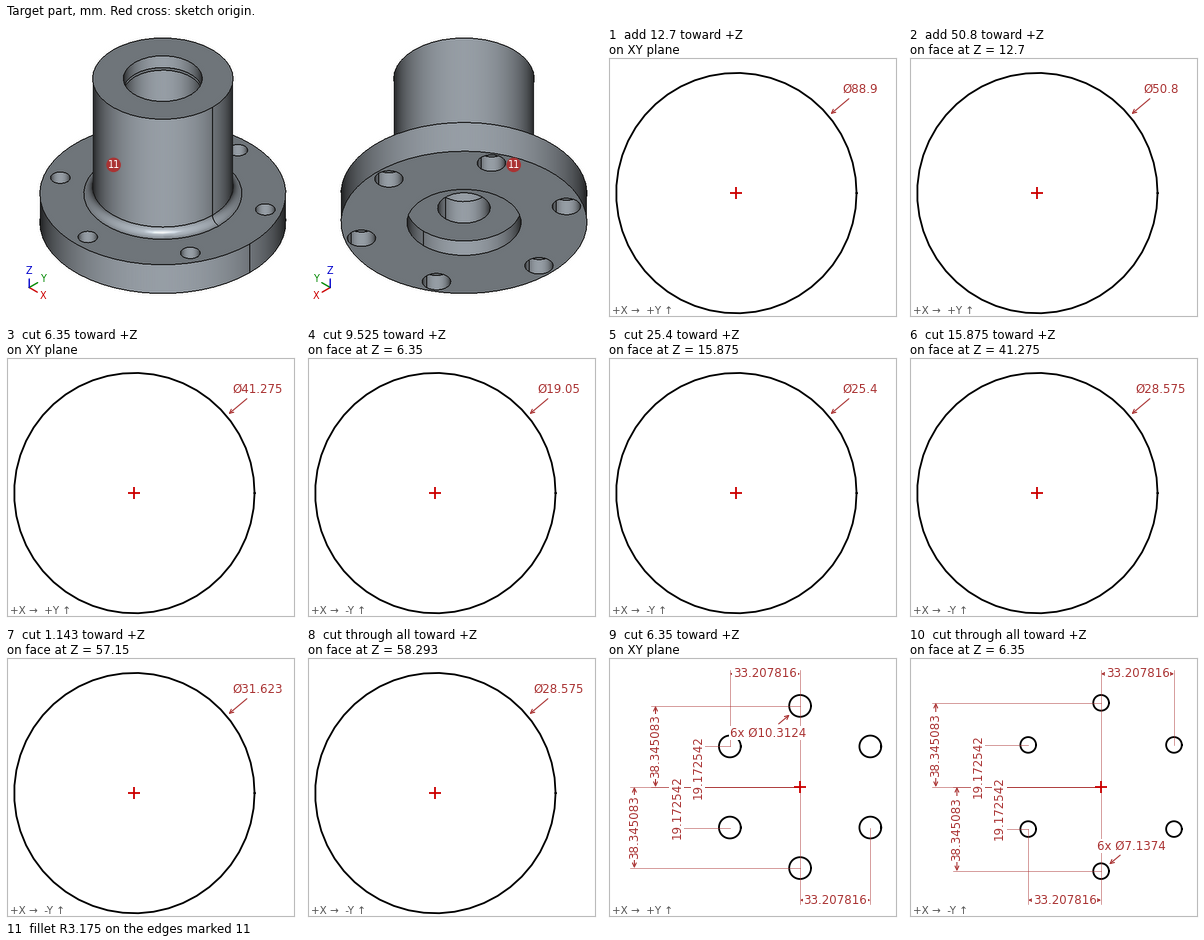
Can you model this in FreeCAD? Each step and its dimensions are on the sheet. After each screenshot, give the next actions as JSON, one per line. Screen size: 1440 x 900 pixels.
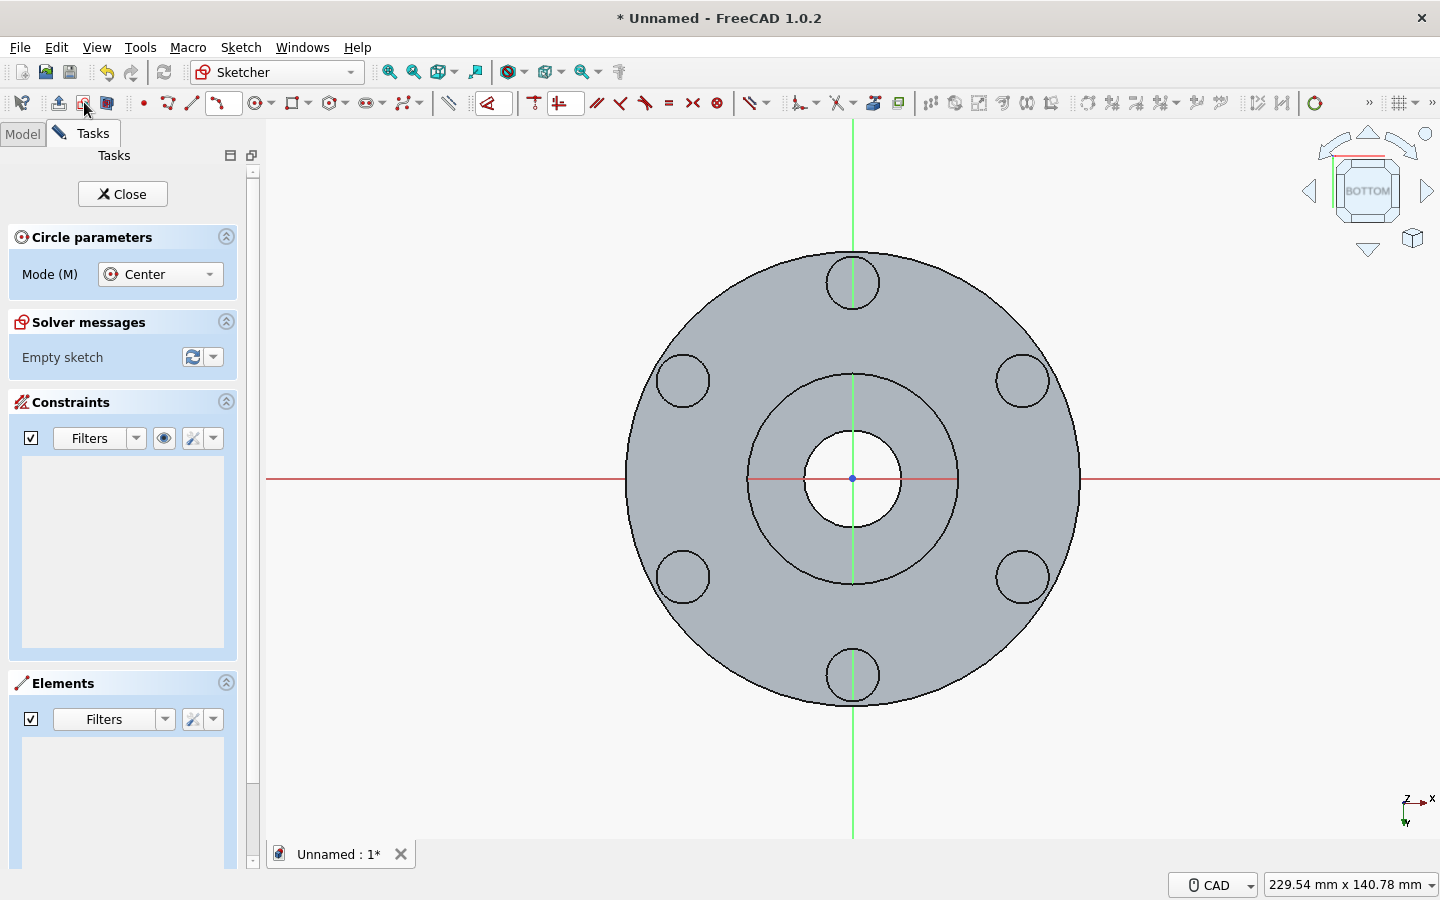
{"action": "scroll", "coordinate": [853, 675], "scroll_direction": "up", "scroll_amount": 2}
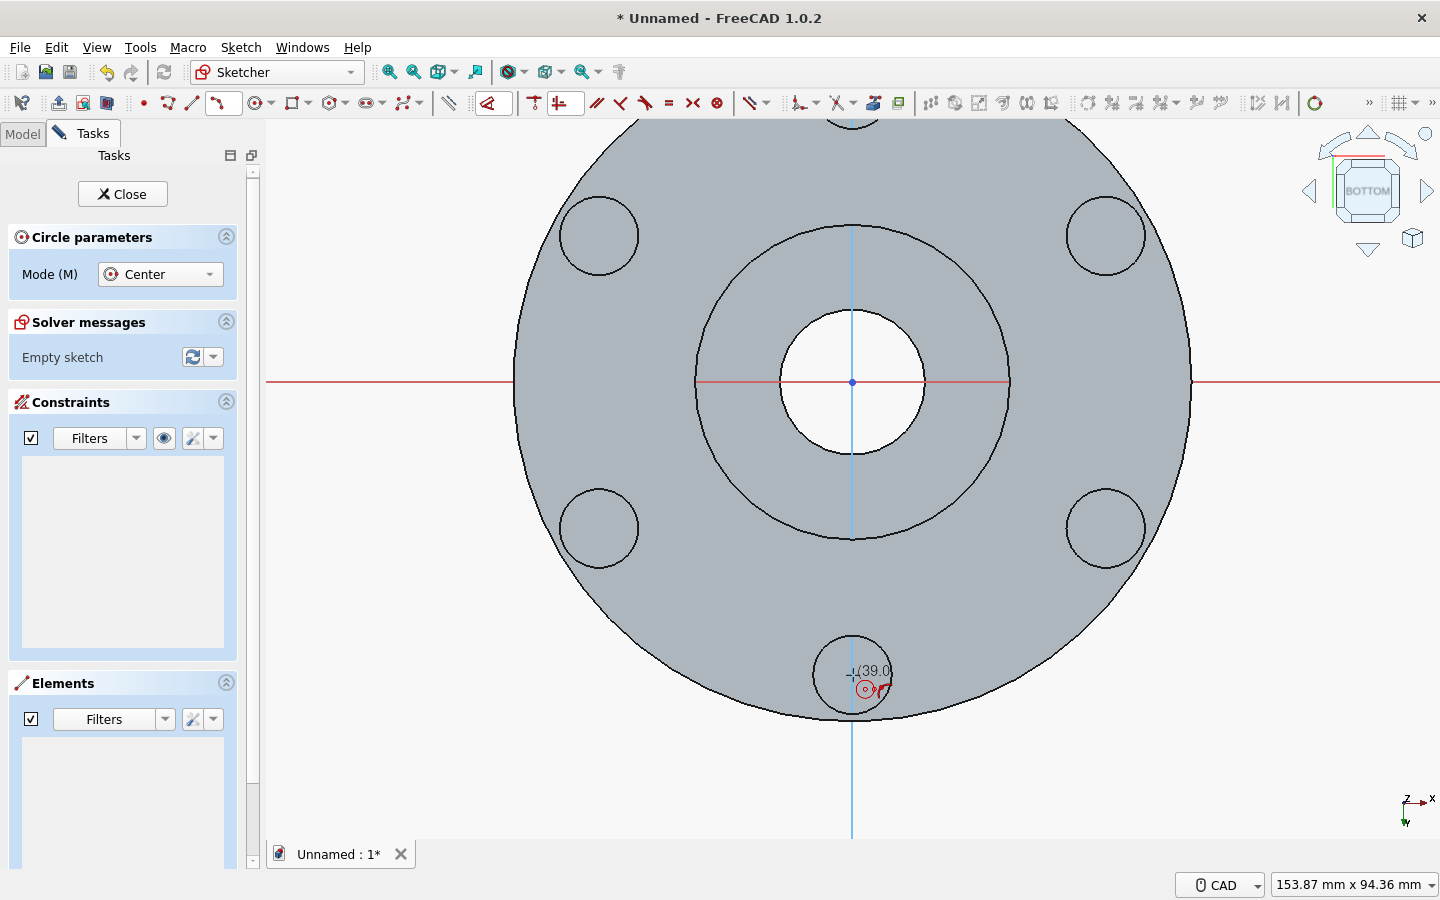
{"action": "left_click", "coordinate": [852, 675]}
{"action": "mouse_move", "coordinate": [872, 656]}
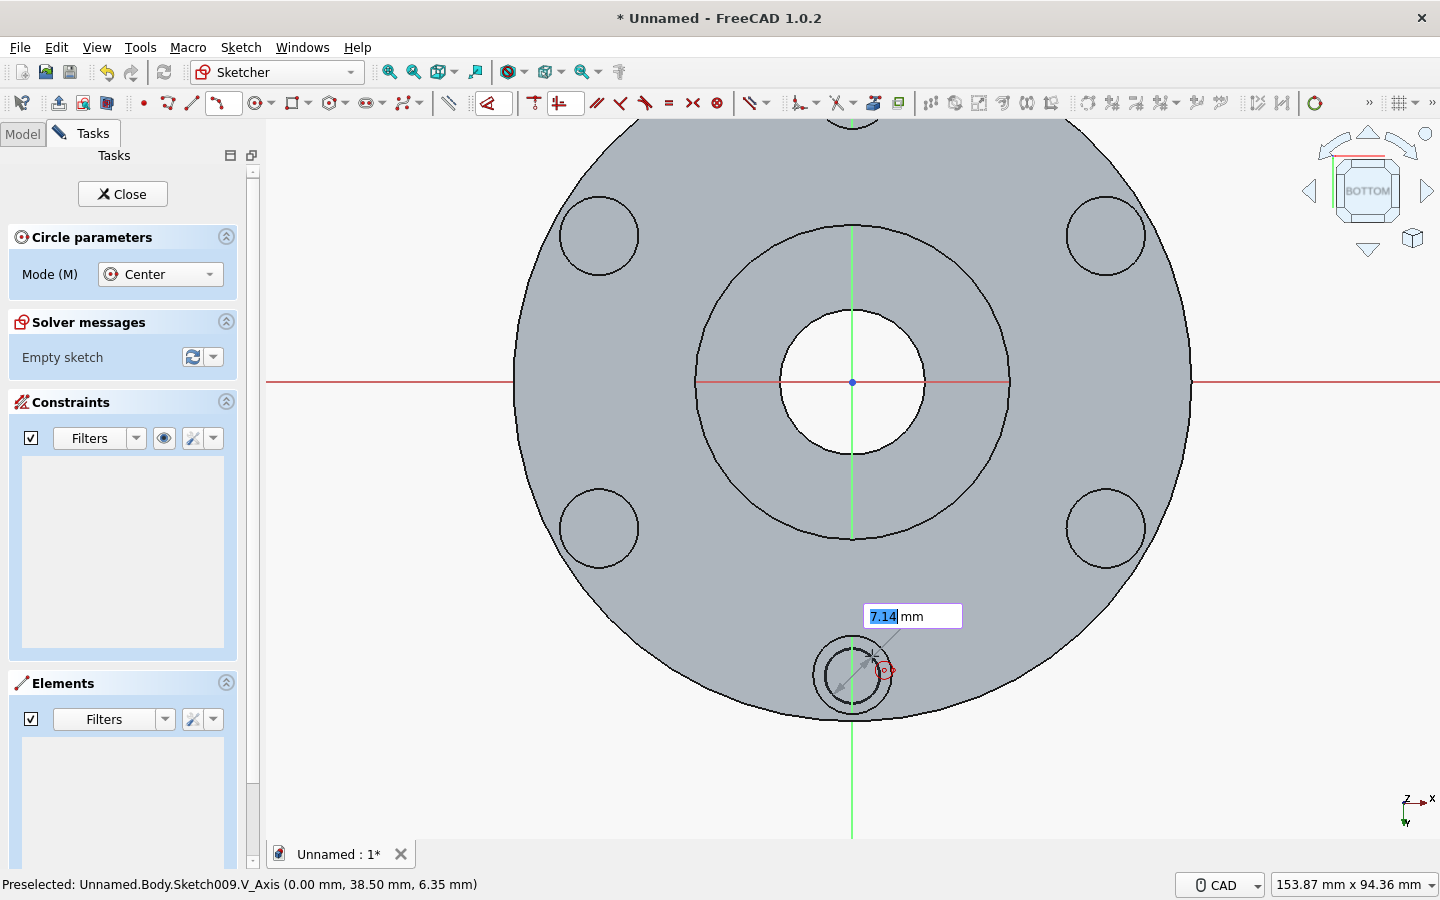
{"action": "type", "text": "7.1374"}
{"action": "key", "text": "Return"}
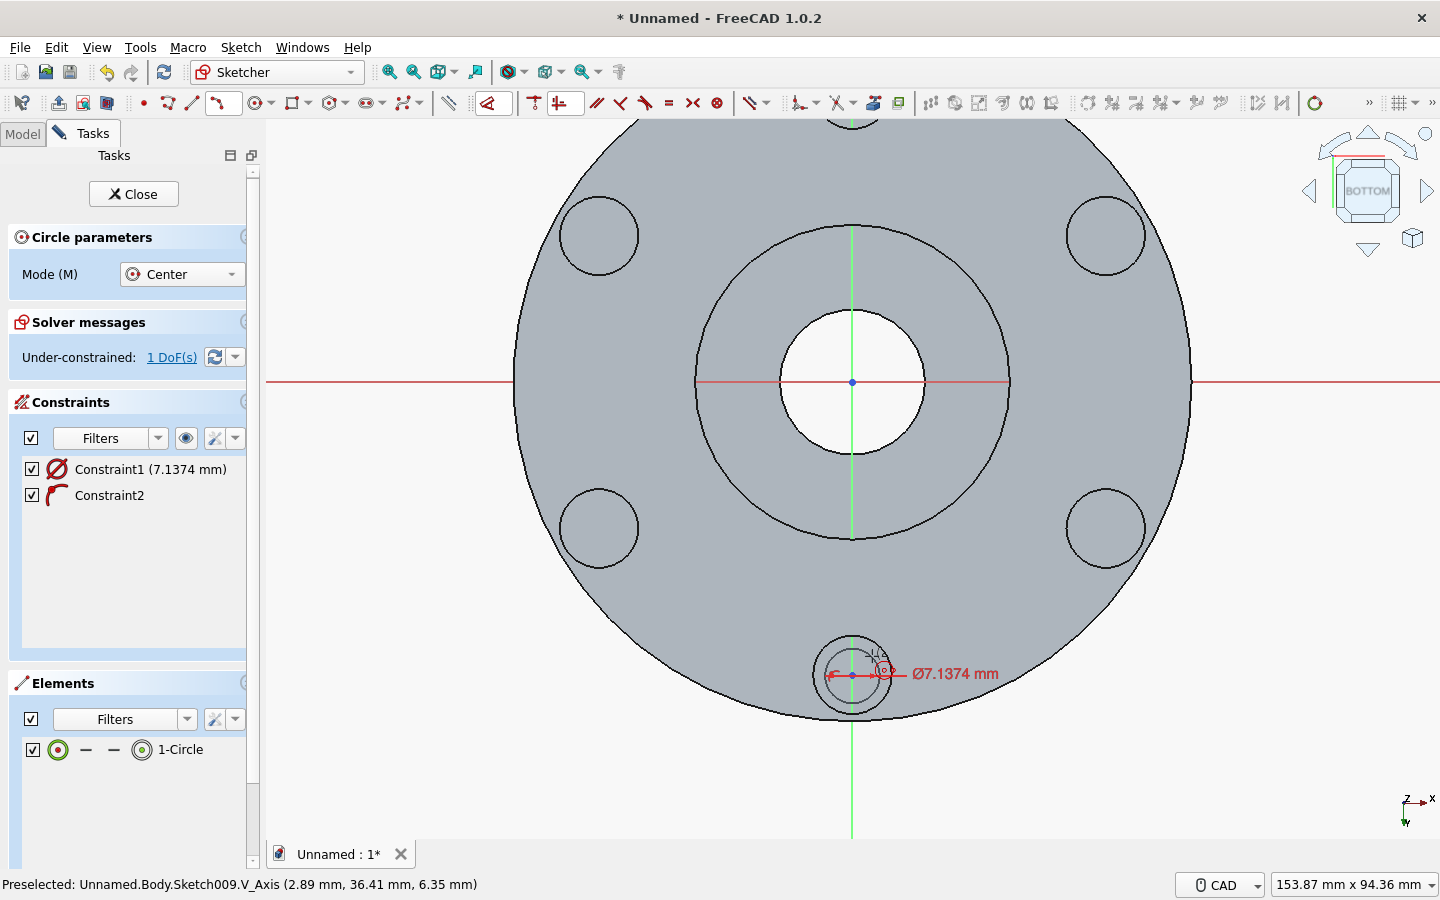
{"action": "left_click", "coordinate": [599, 529]}
{"action": "mouse_move", "coordinate": [618, 509]}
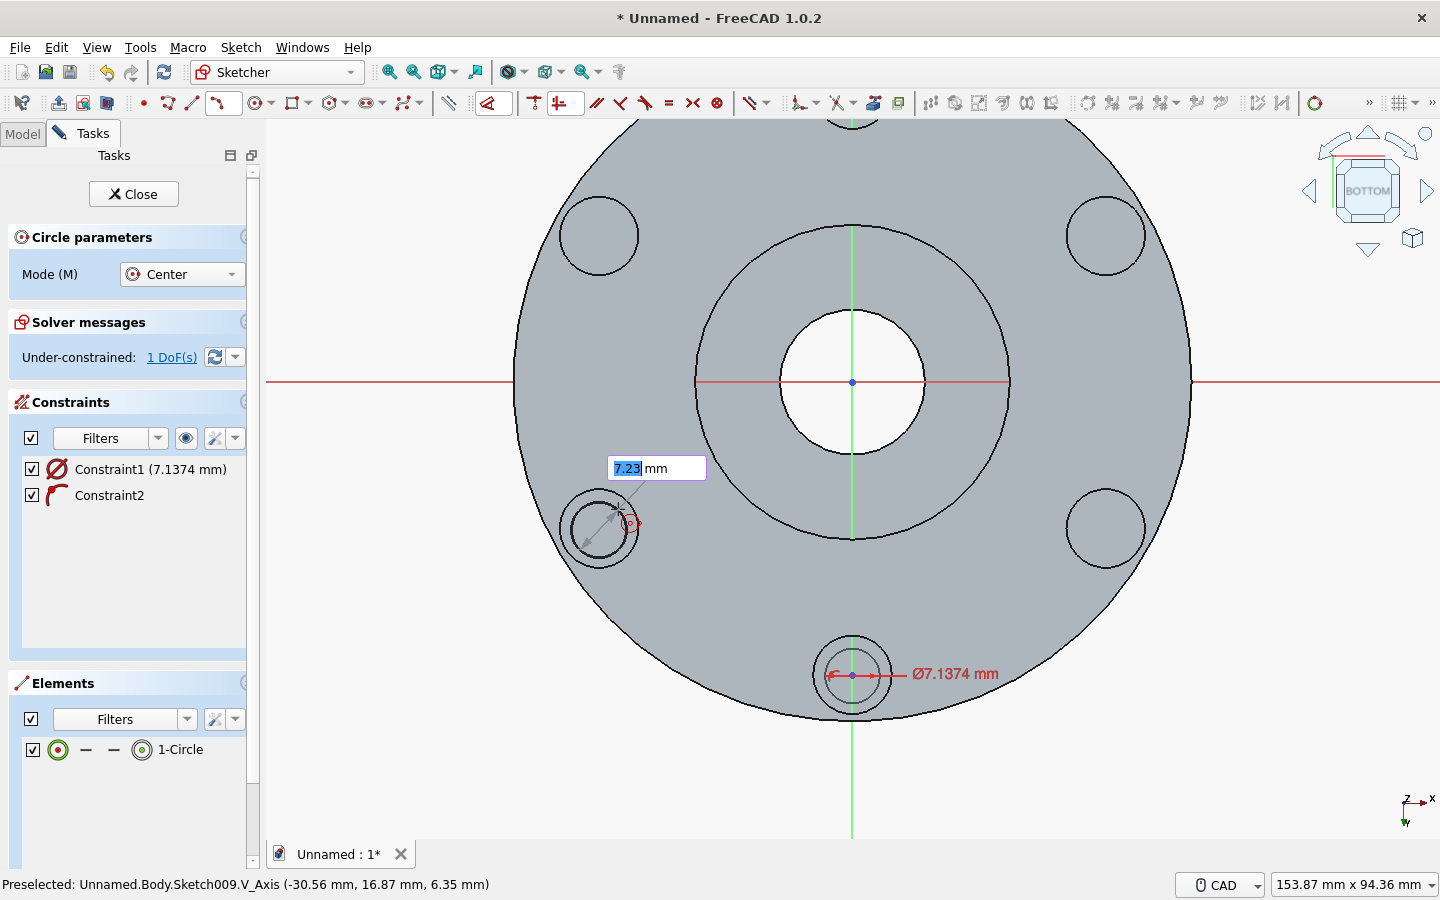
{"action": "type", "text": "7.1374"}
{"action": "key", "text": "Return"}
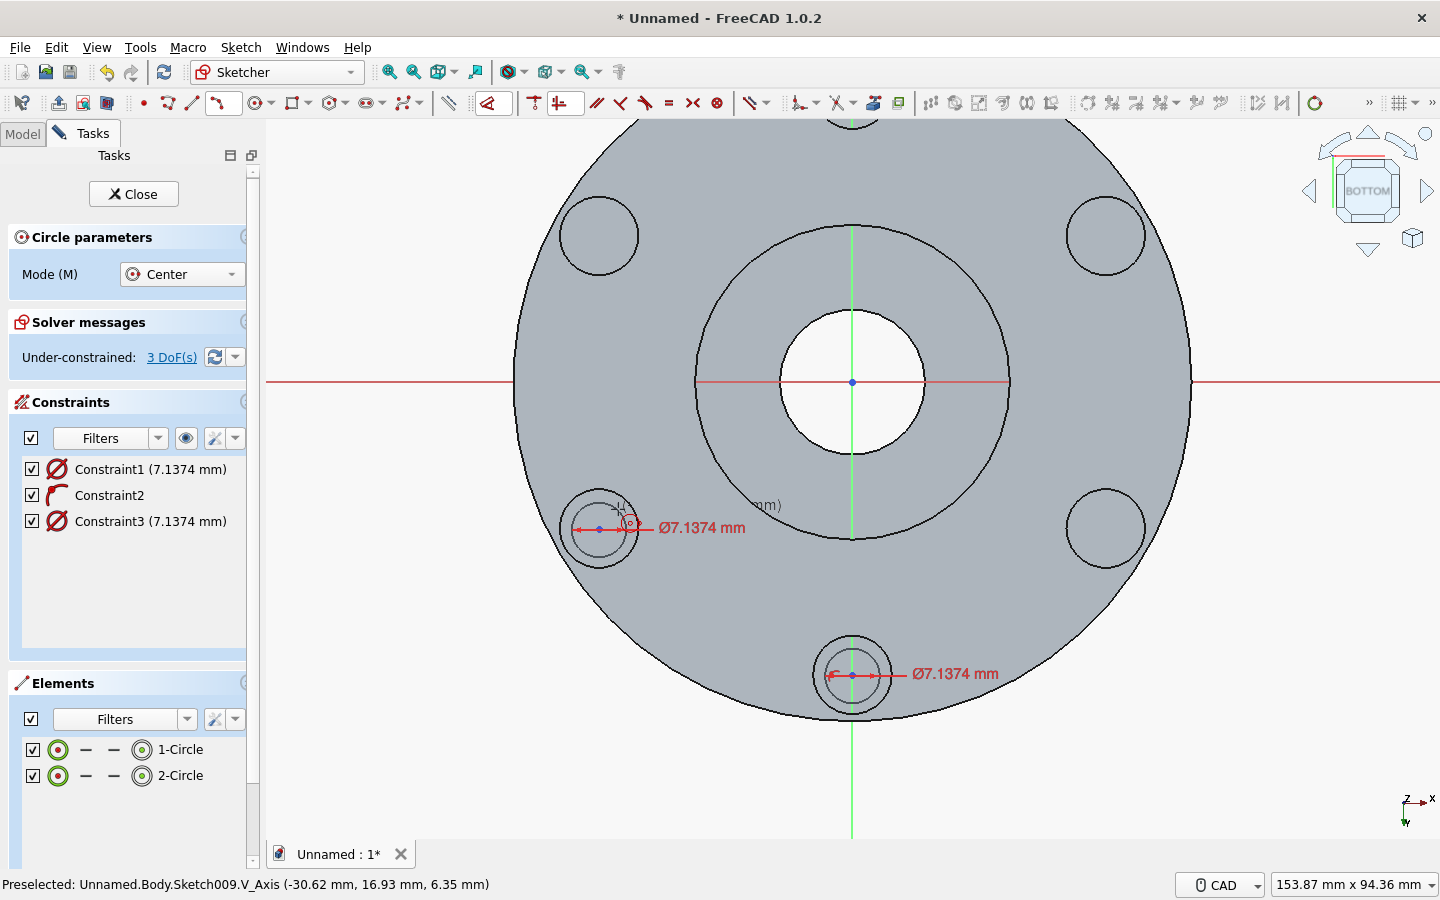
{"action": "left_click", "coordinate": [599, 236]}
{"action": "mouse_move", "coordinate": [618, 217]}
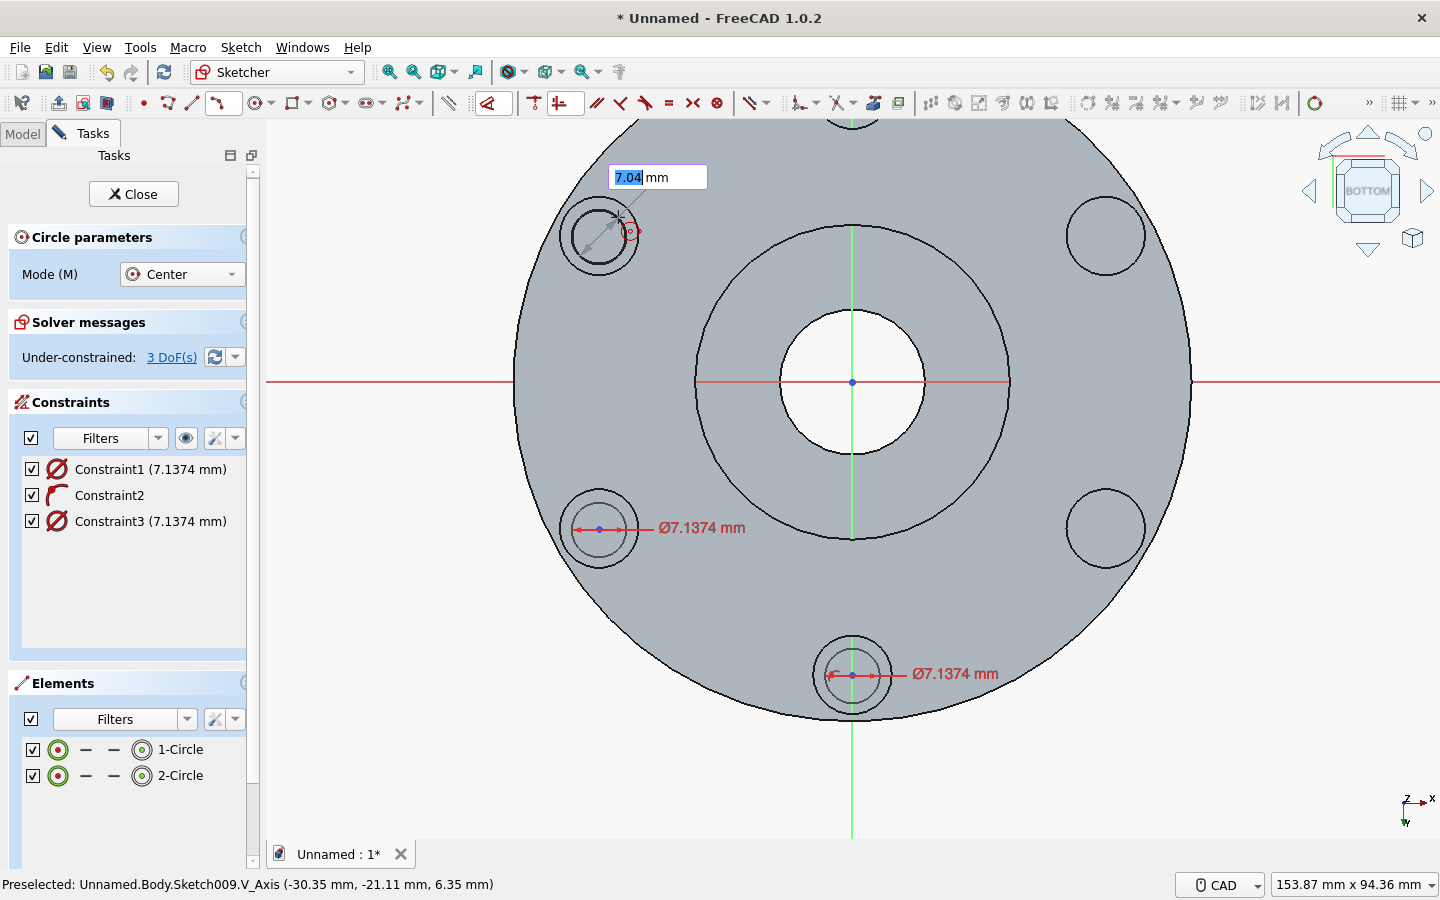
{"action": "type", "text": "7.1374"}
{"action": "key", "text": "Return"}